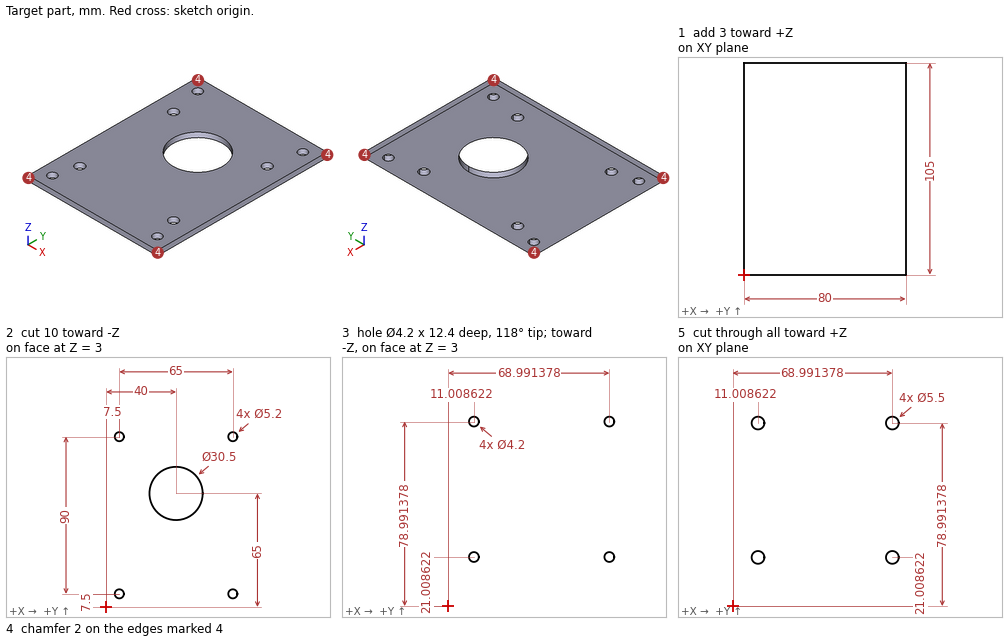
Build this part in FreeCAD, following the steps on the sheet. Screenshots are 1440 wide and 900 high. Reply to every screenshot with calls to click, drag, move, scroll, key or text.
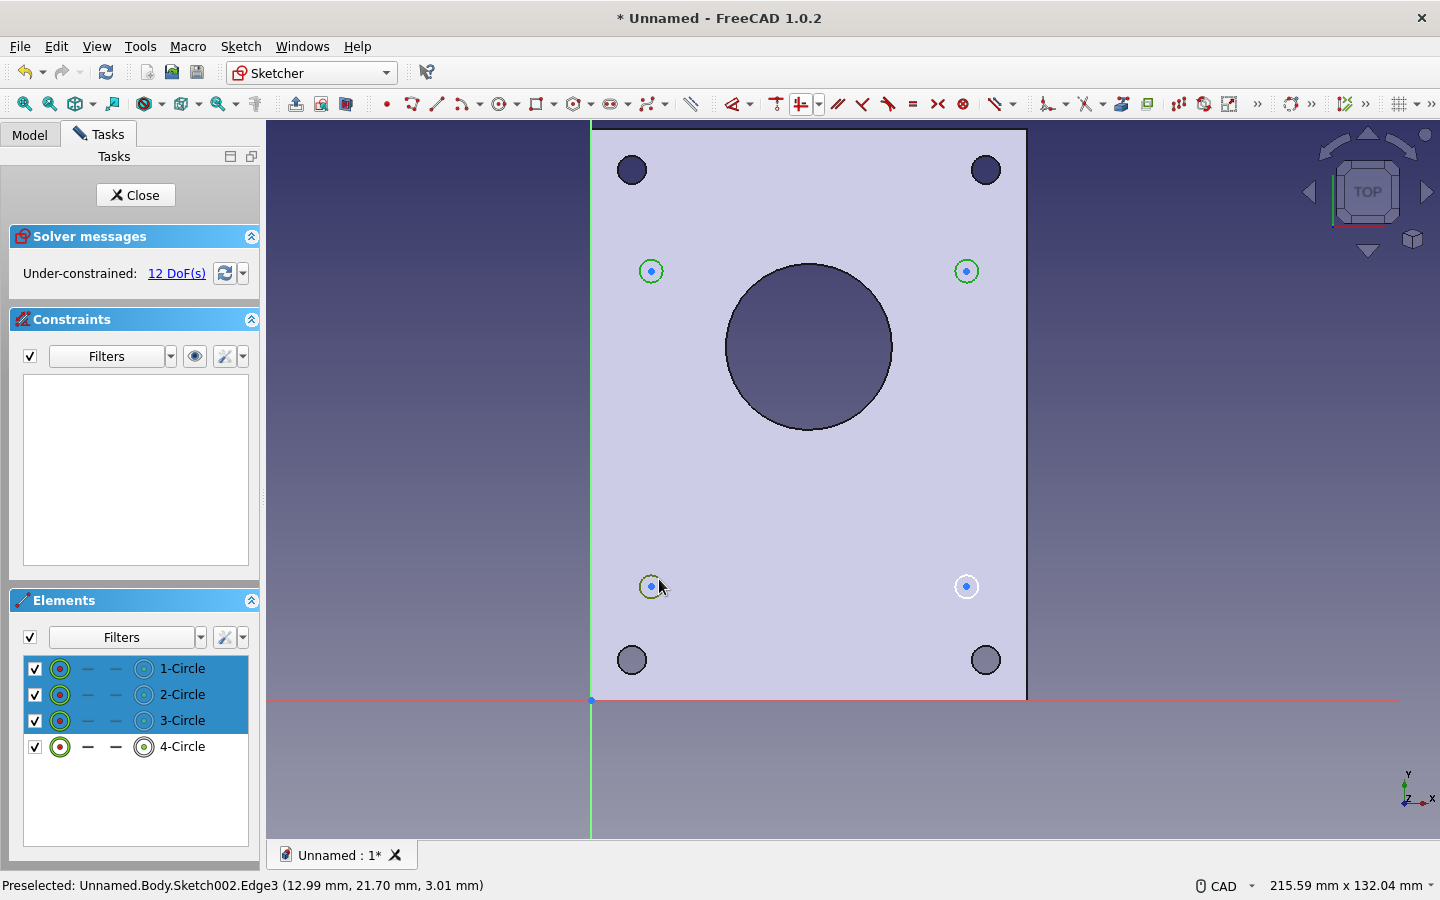
click(975, 579)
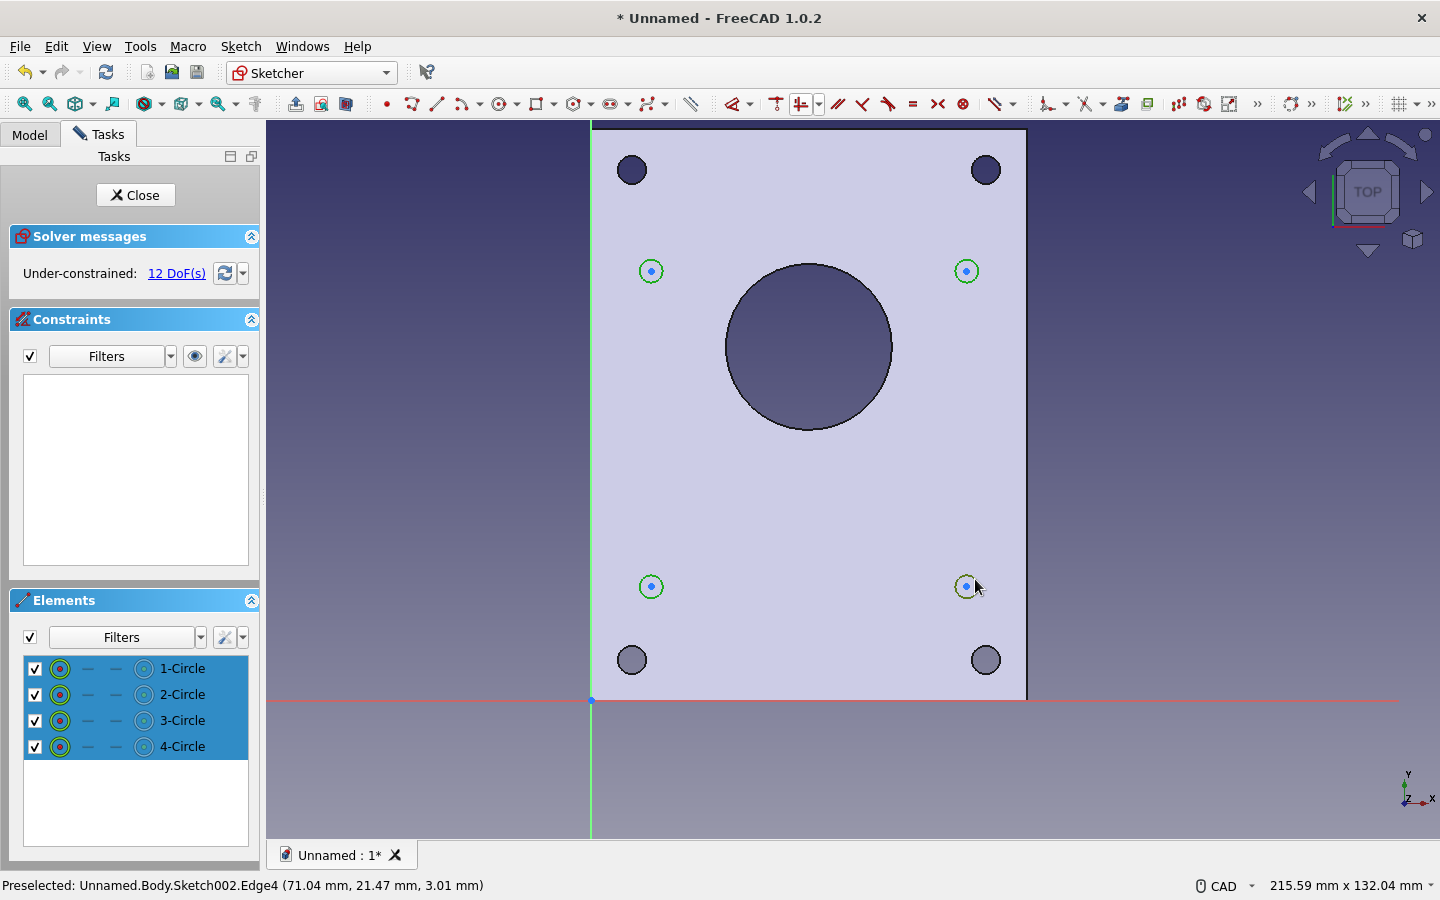
click(913, 104)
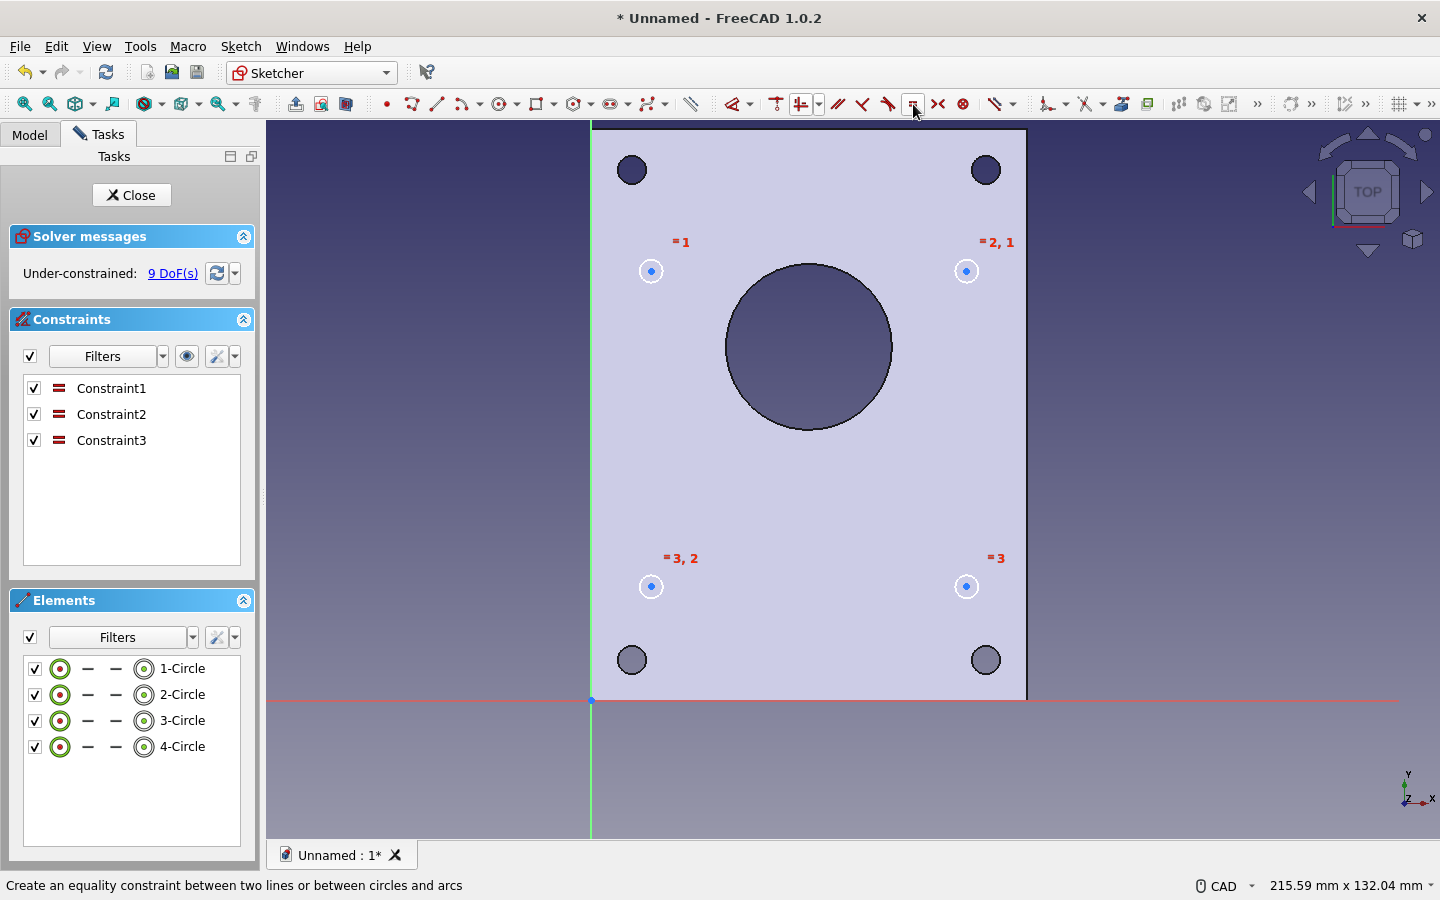
click(651, 271)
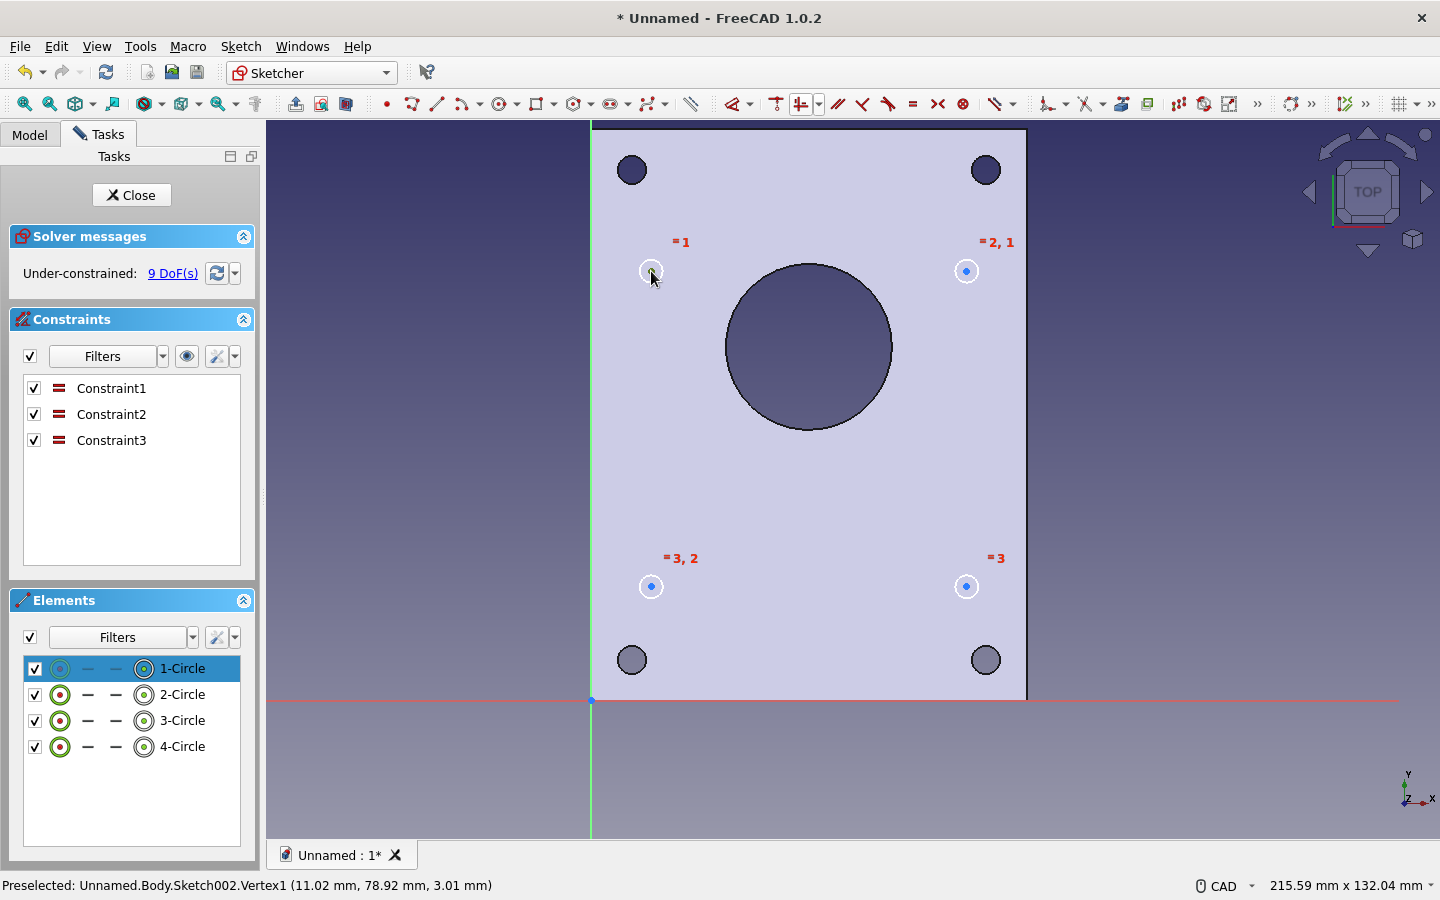
click(967, 271)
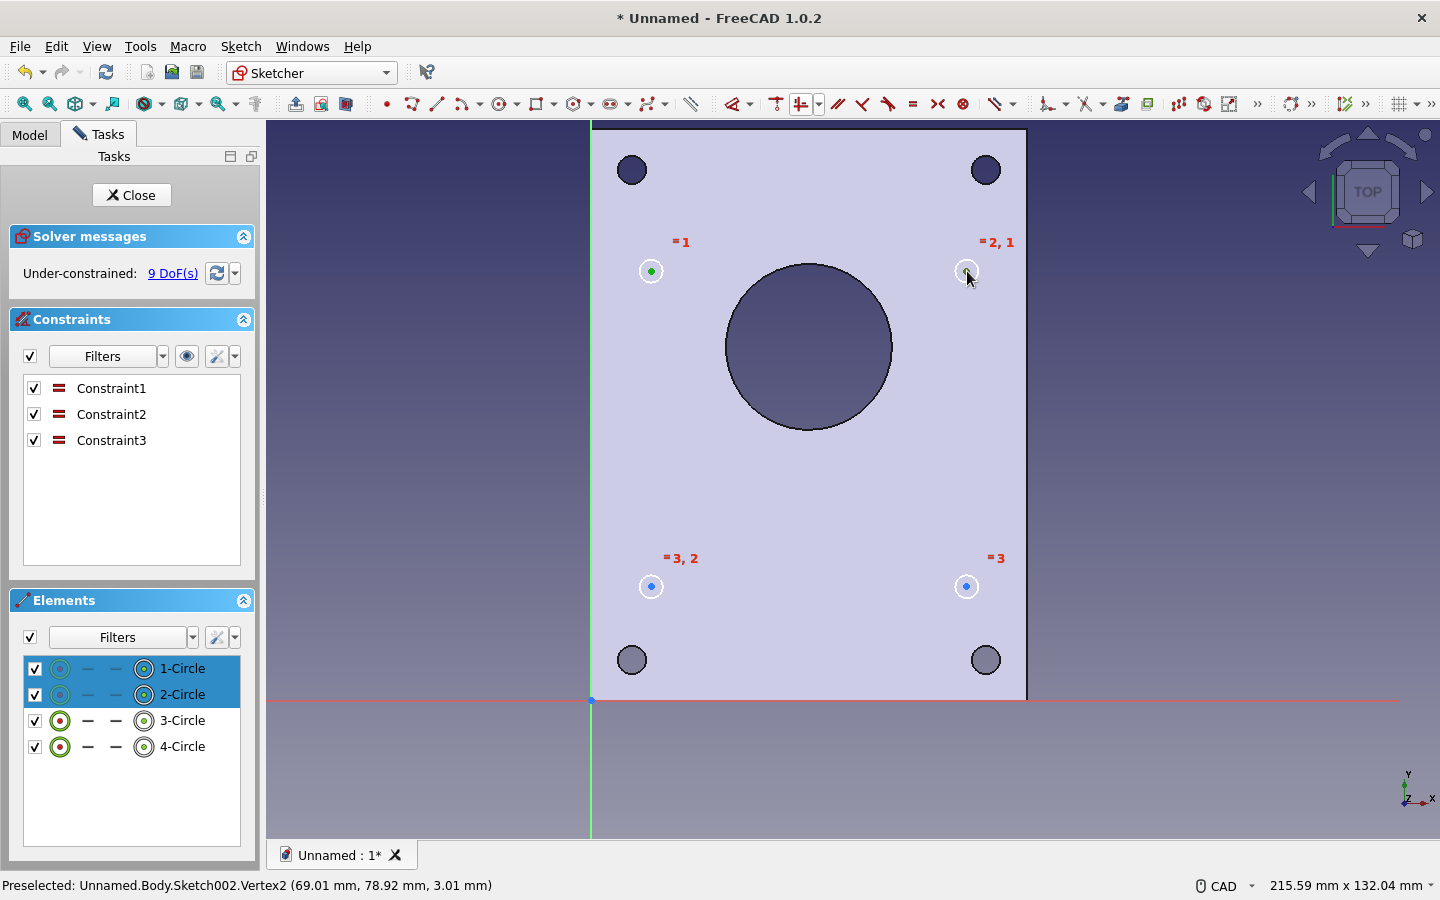
key(h)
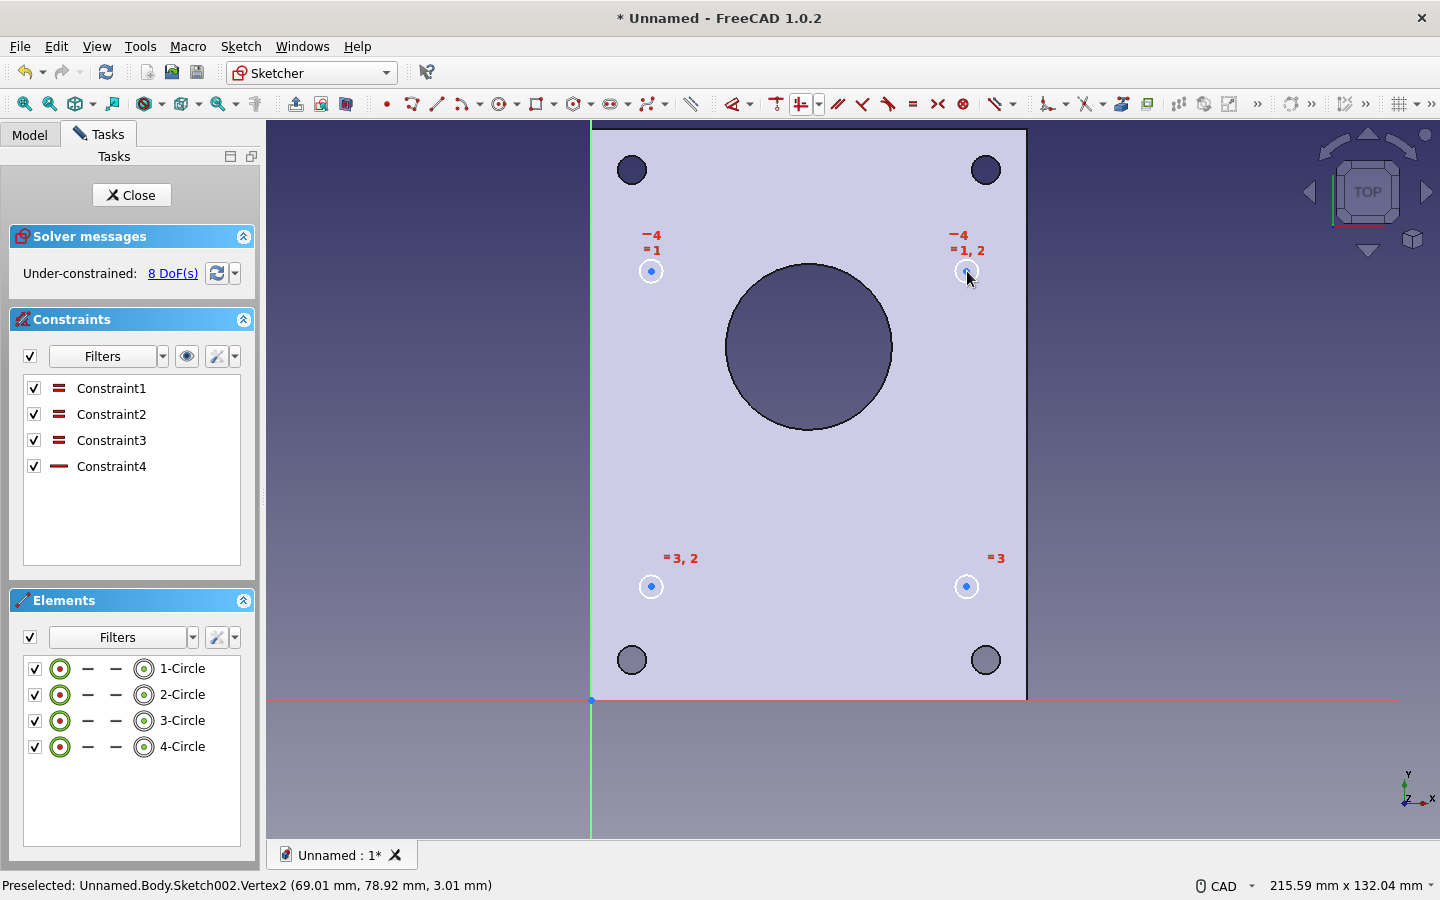
click(651, 271)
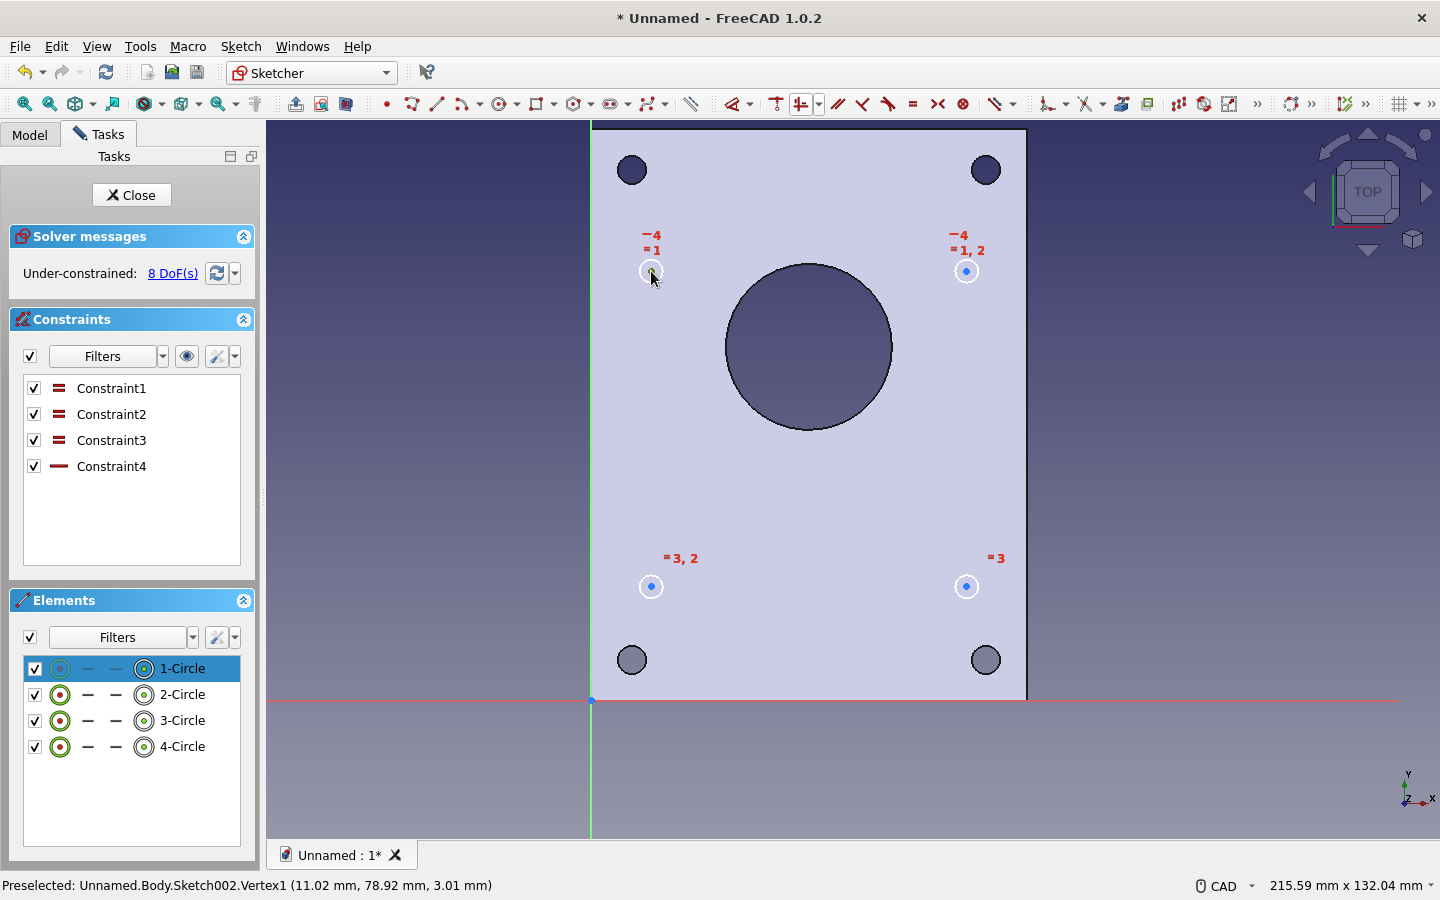
click(651, 587)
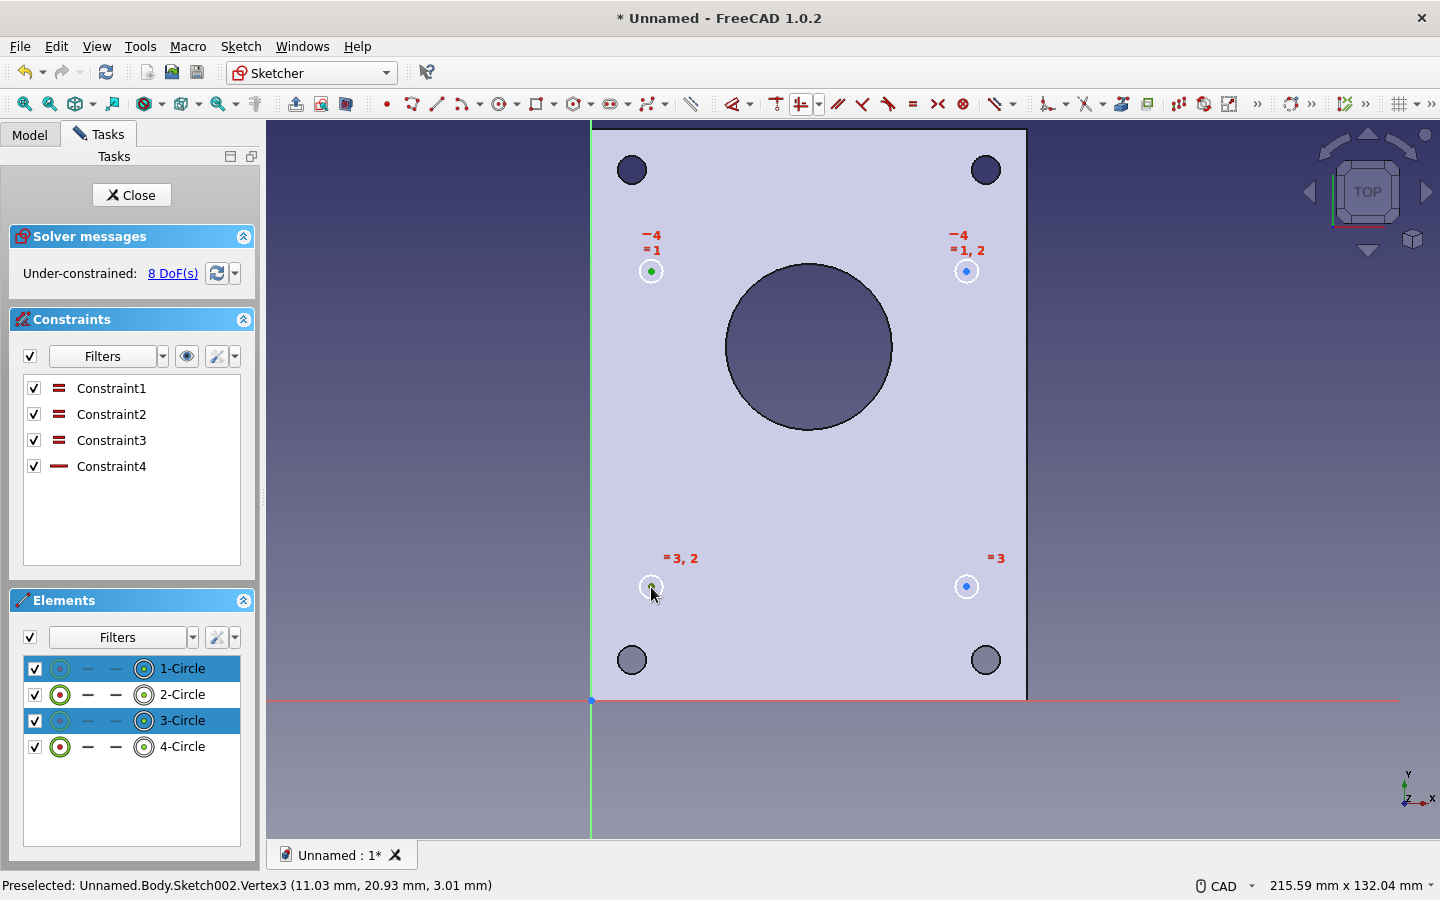
click(818, 104)